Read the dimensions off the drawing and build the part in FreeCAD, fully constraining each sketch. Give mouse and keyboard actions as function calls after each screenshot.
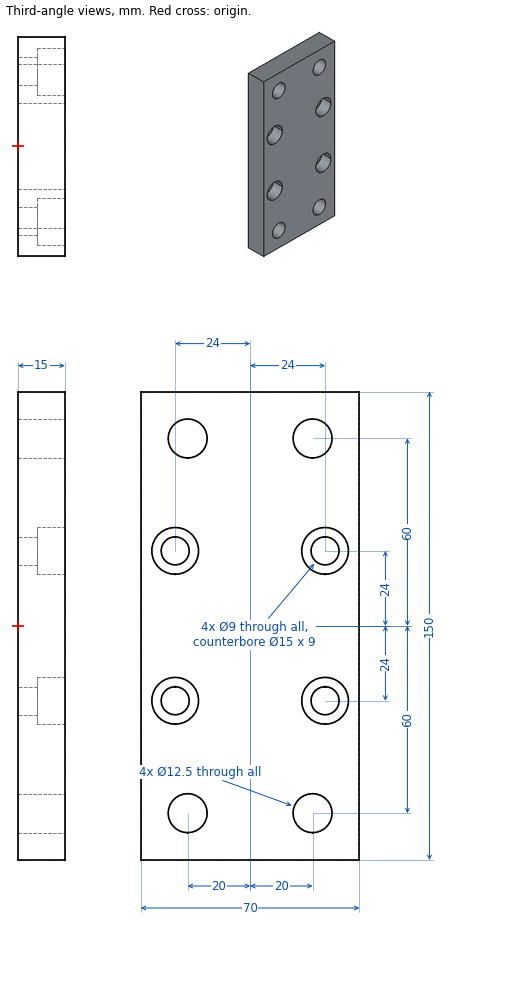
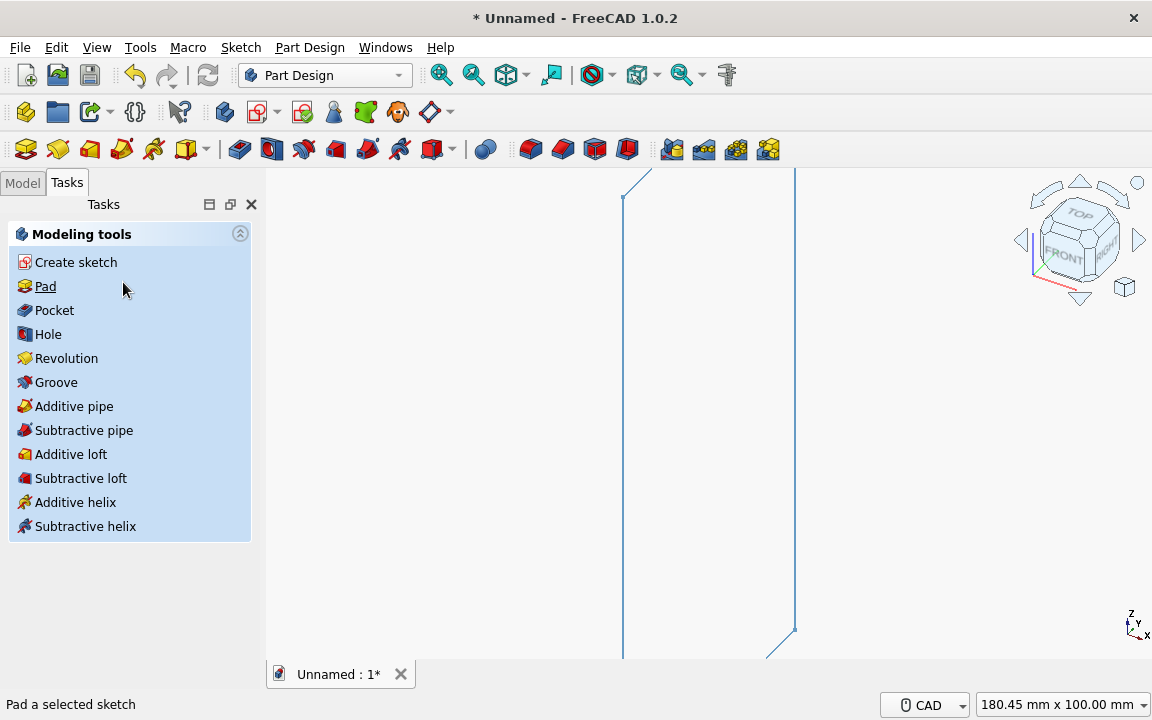
click(26, 150)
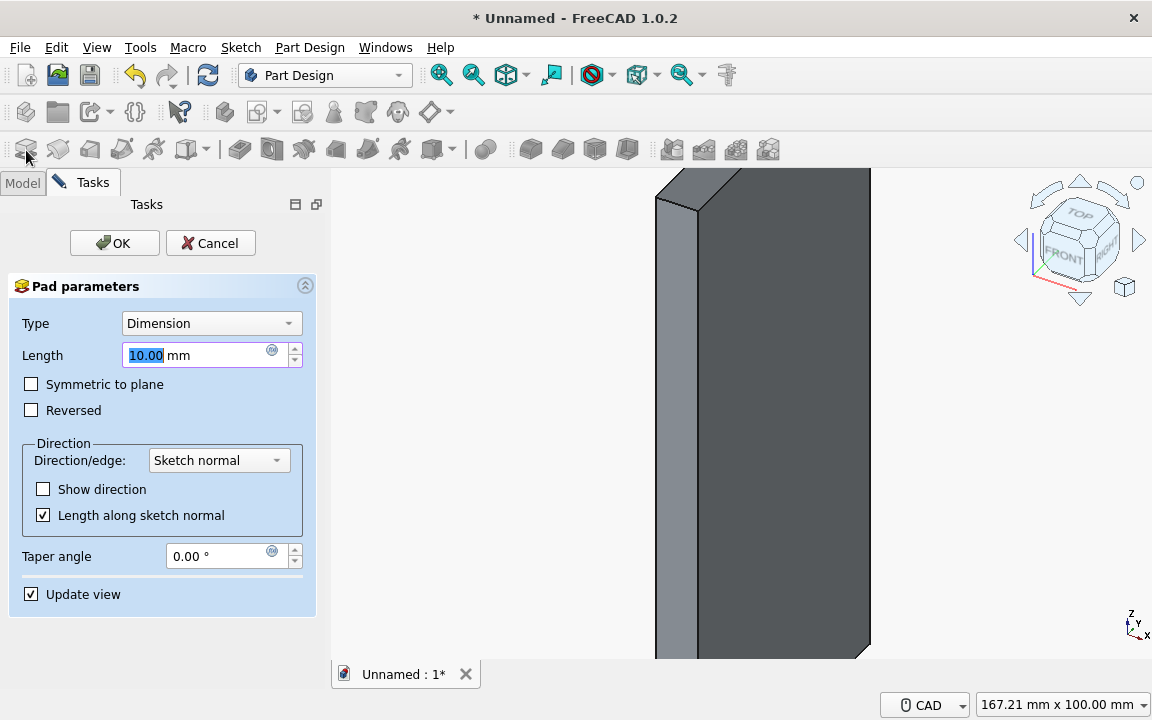
text(15)
key(Tab)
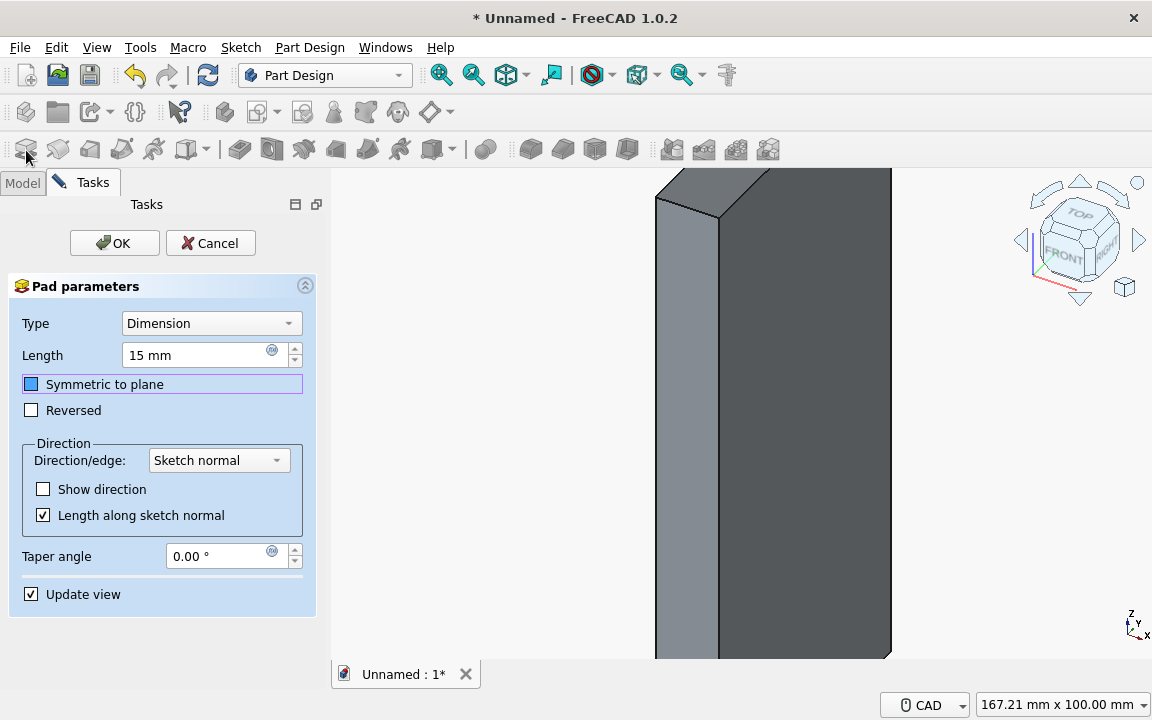
click(115, 243)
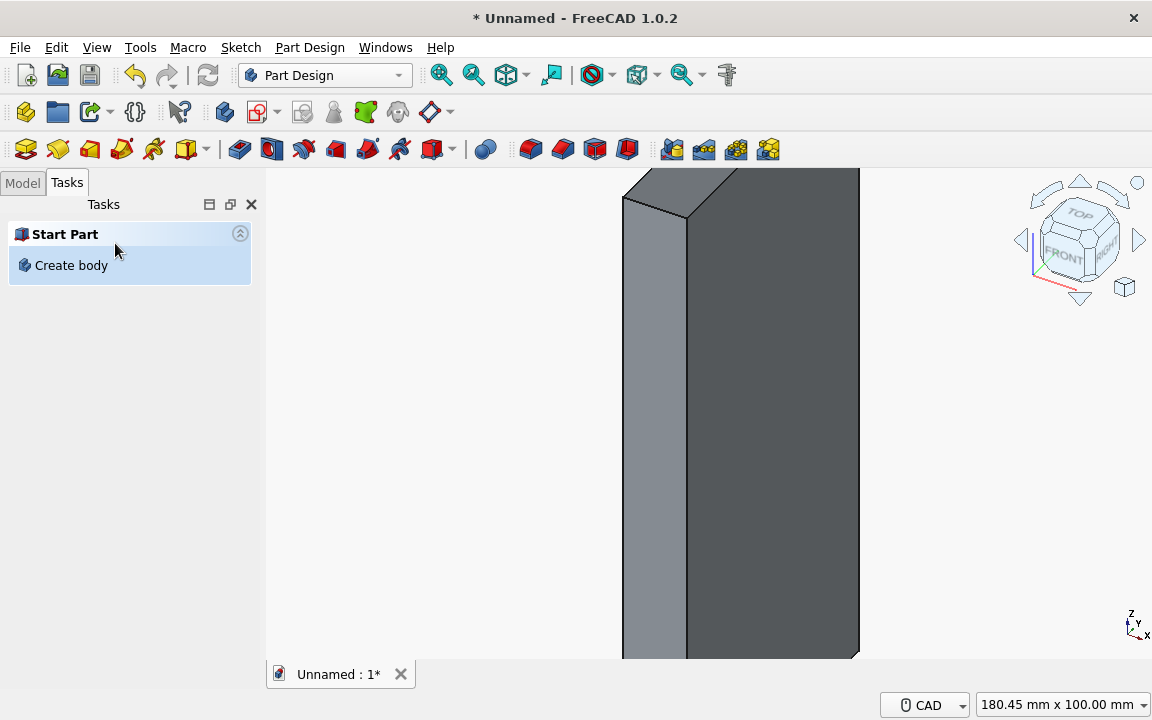
click(442, 76)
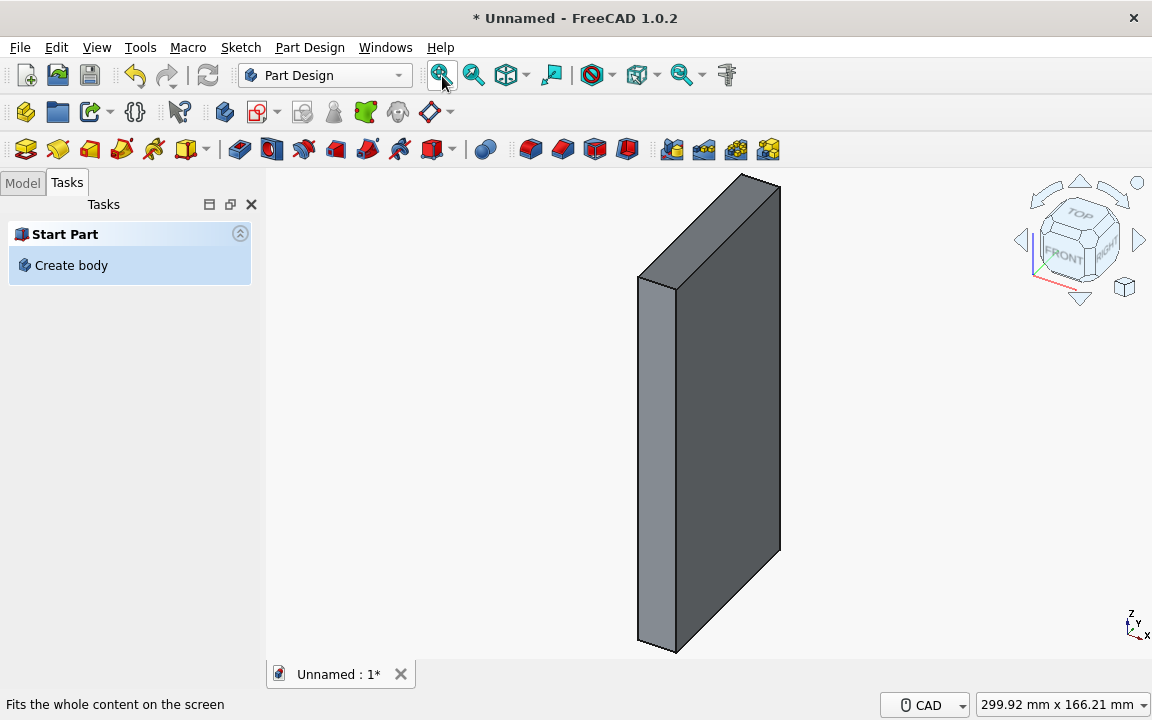
click(728, 471)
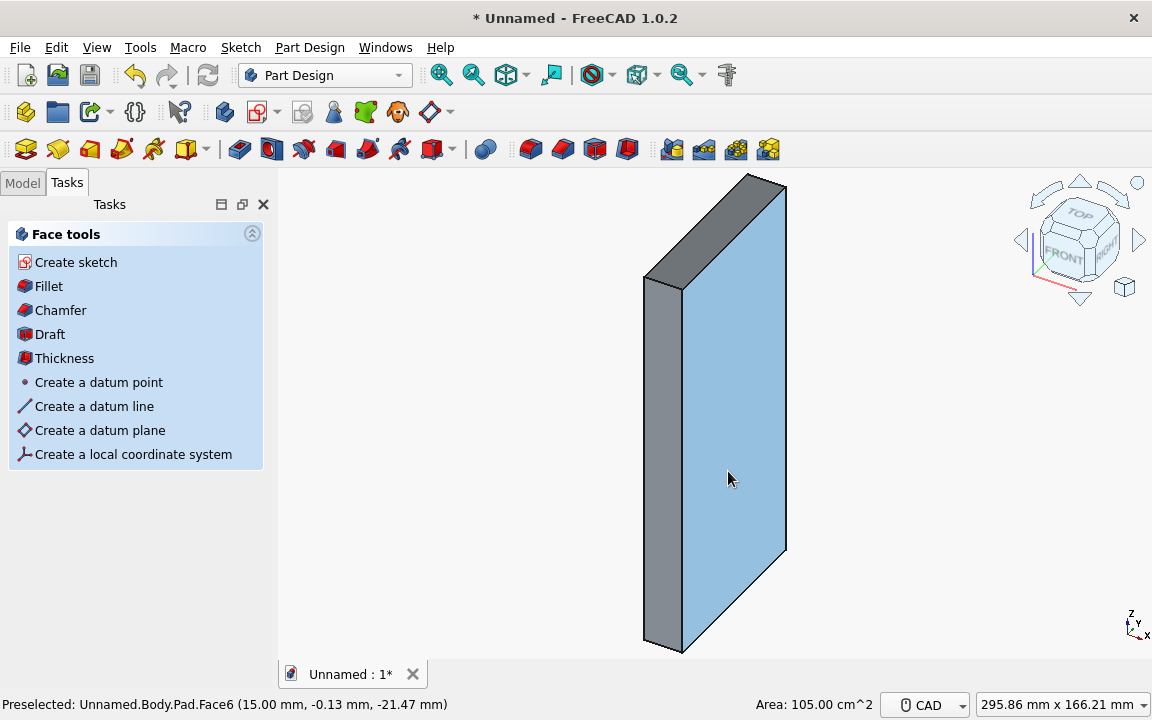
click(258, 112)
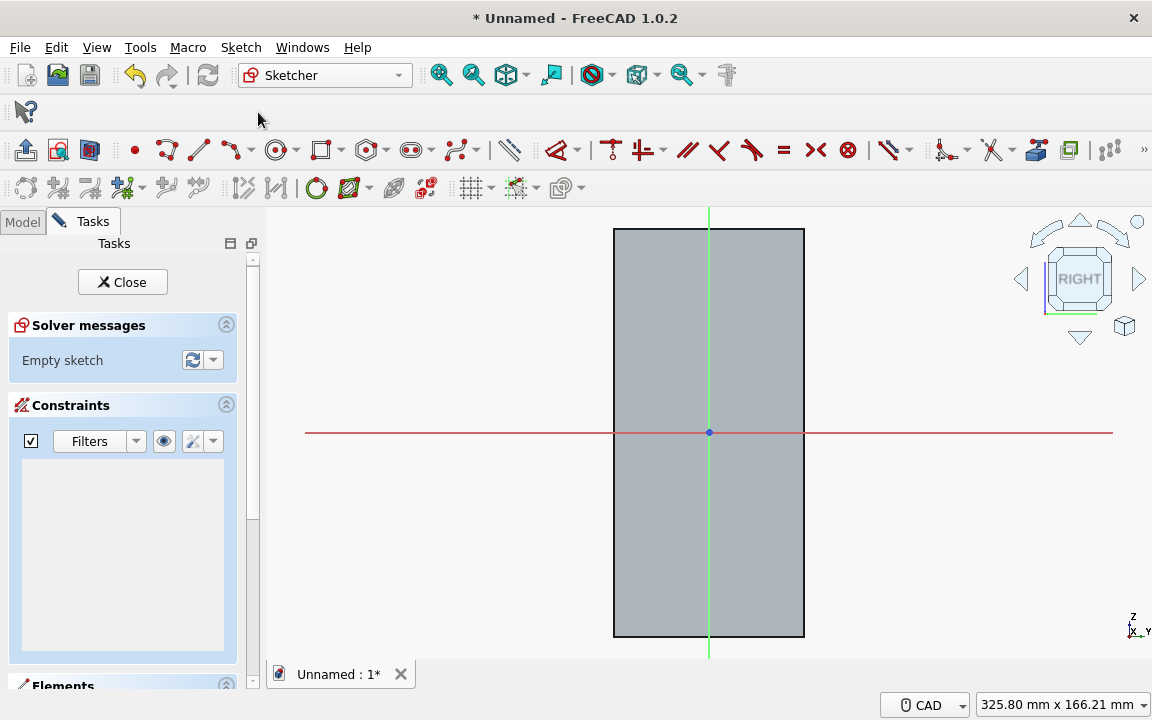
scroll(792, 433, up, 3)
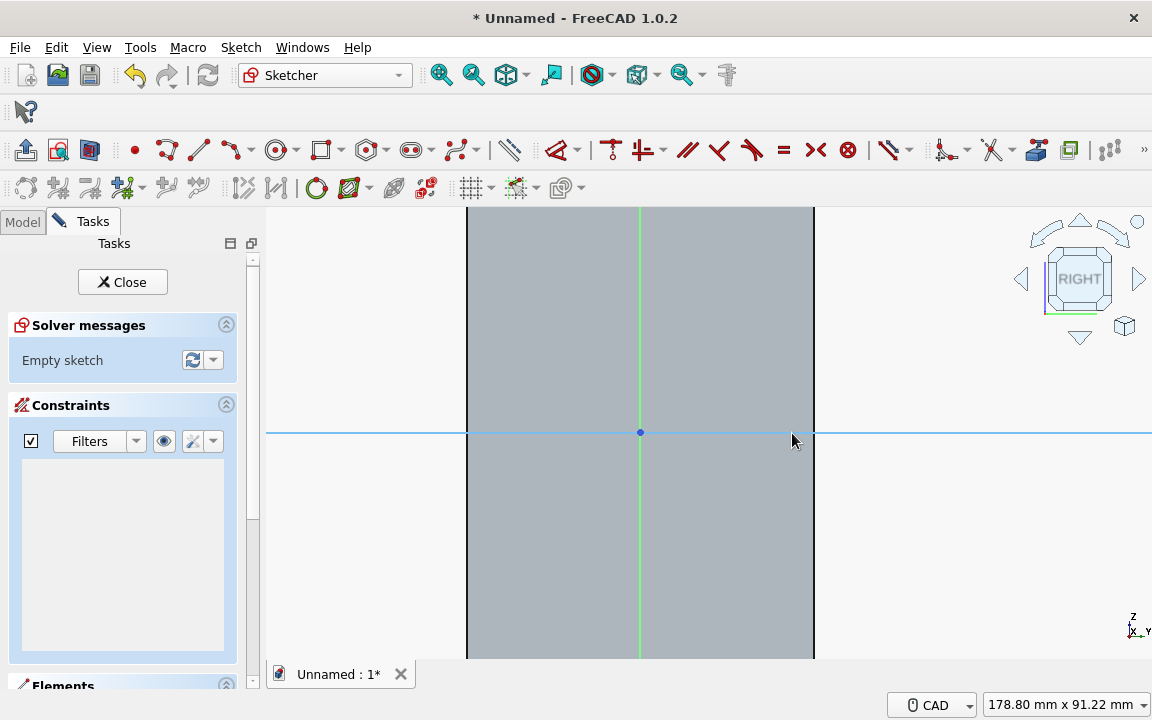
click(276, 150)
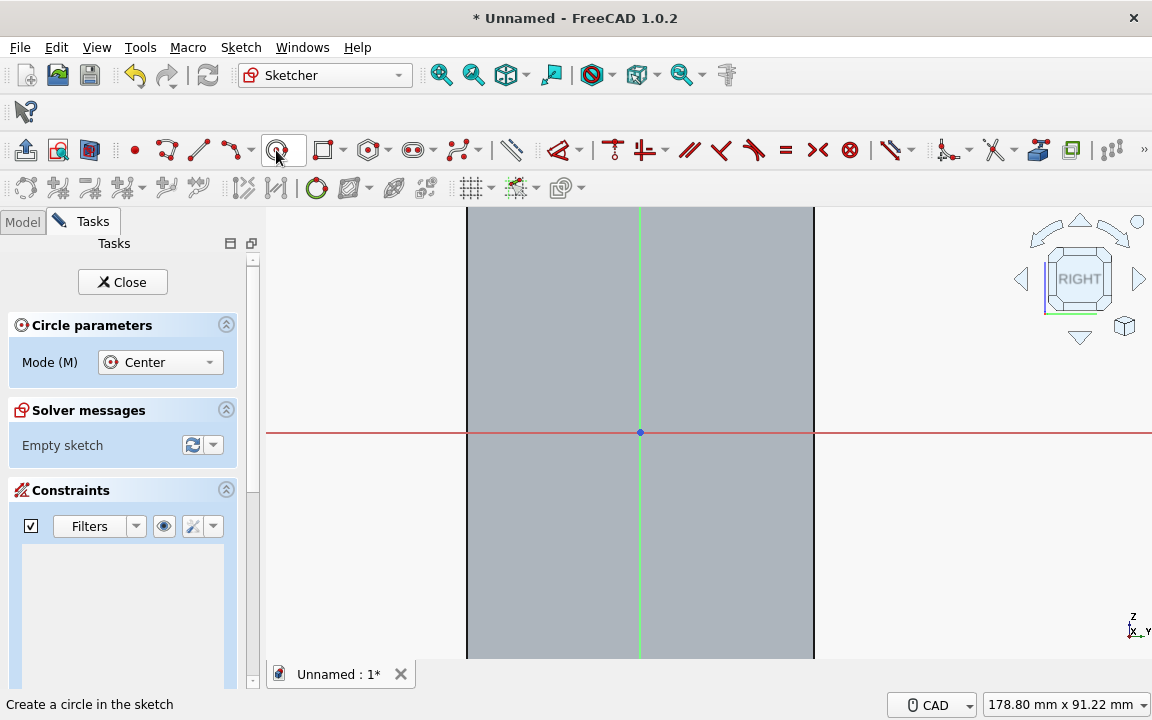
click(759, 314)
click(775, 298)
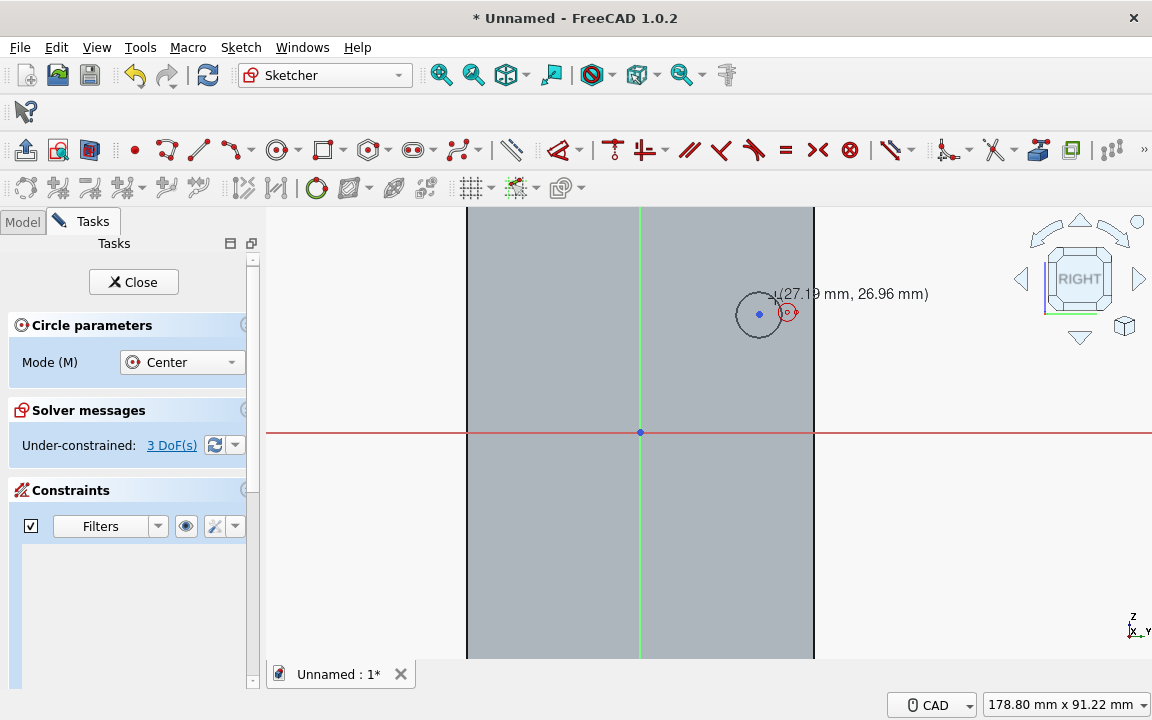
click(759, 552)
click(775, 536)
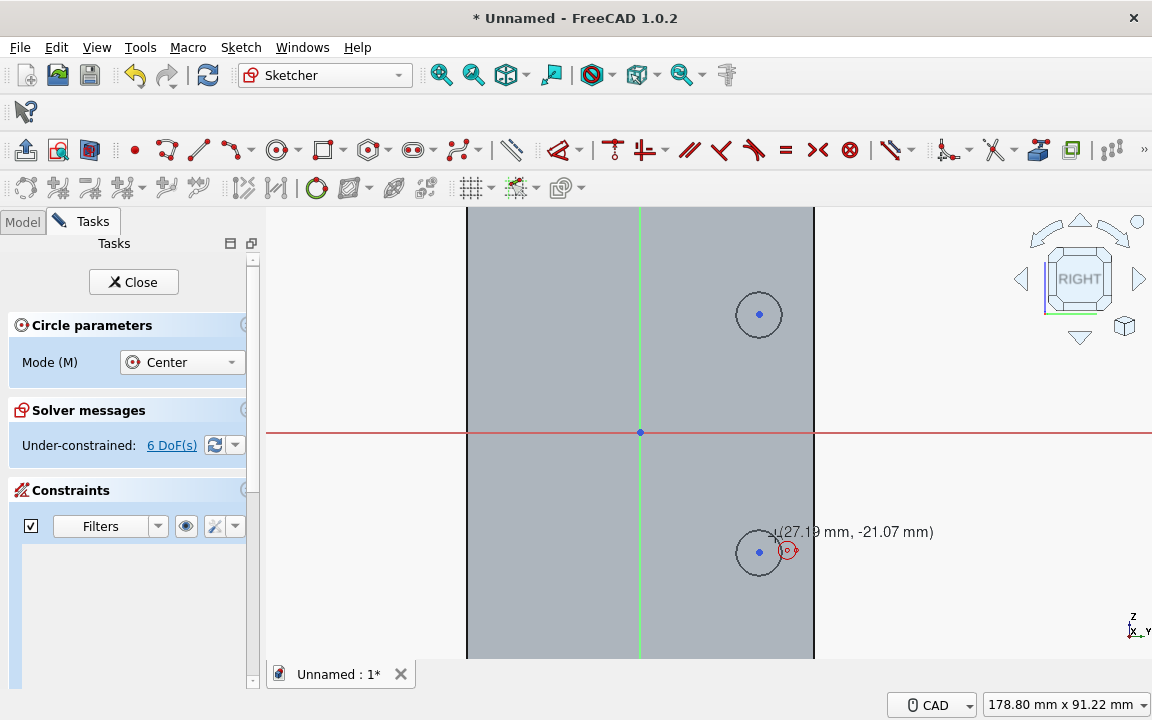
click(521, 314)
click(537, 298)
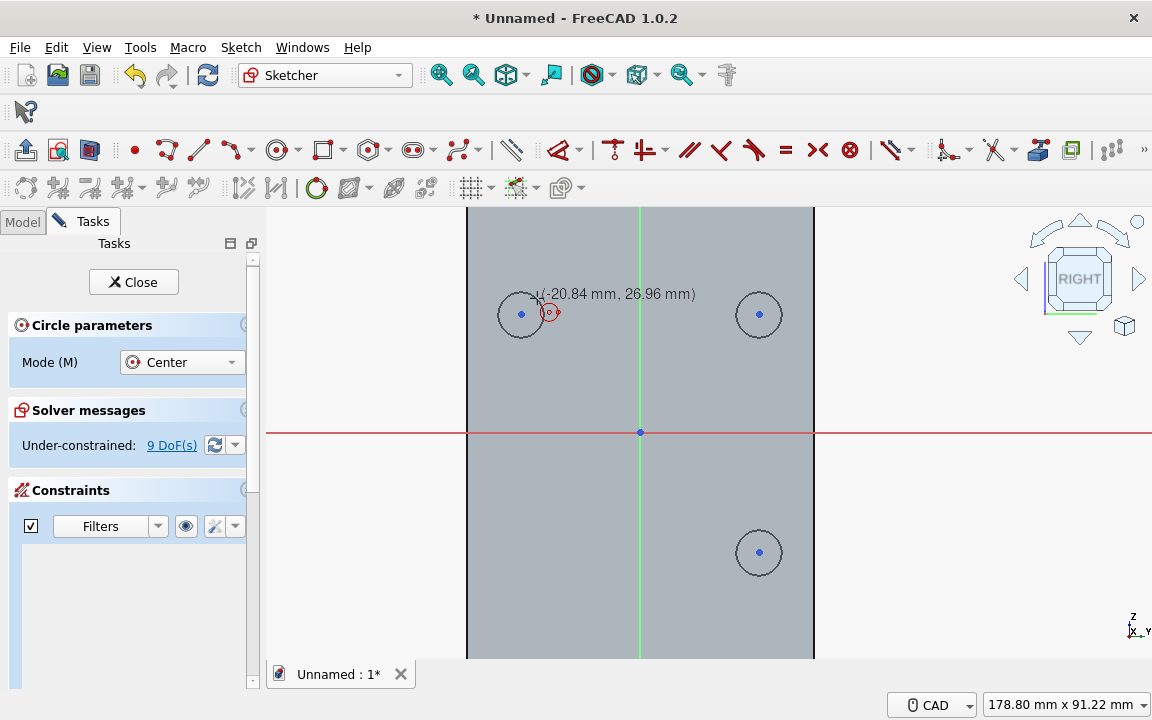
click(521, 552)
click(537, 536)
key(Escape)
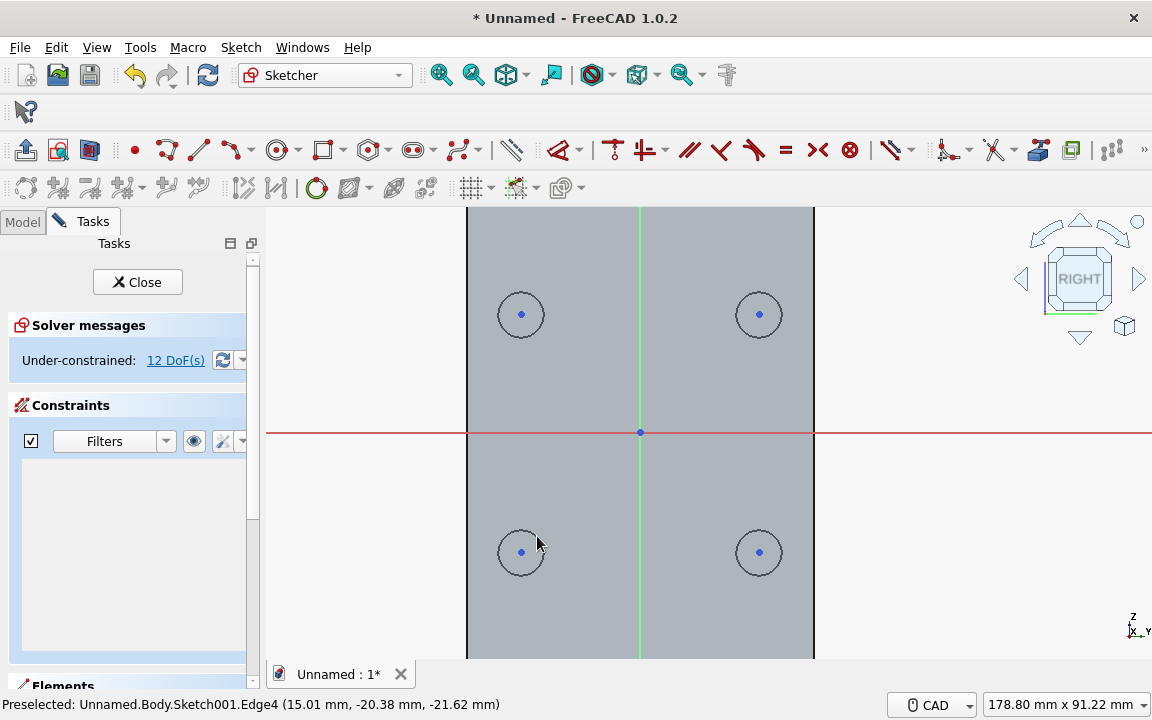
click(775, 299)